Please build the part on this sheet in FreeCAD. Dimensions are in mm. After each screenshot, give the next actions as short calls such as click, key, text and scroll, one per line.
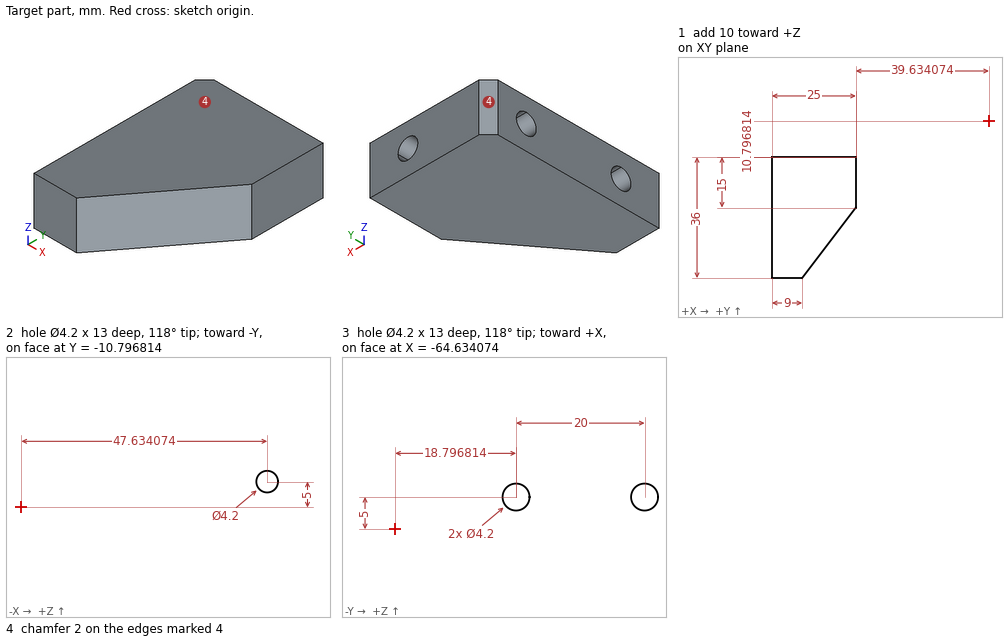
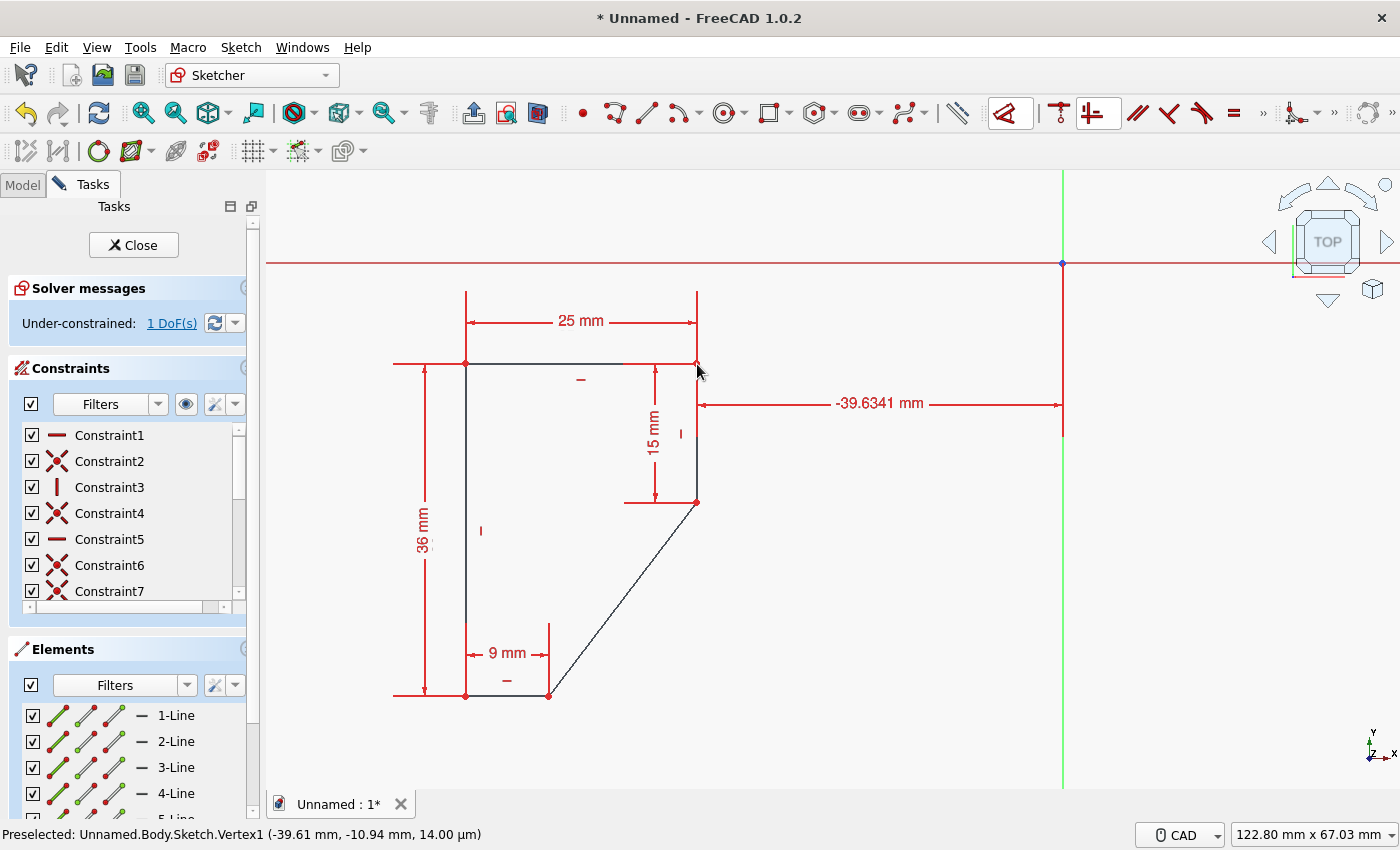
click(697, 364)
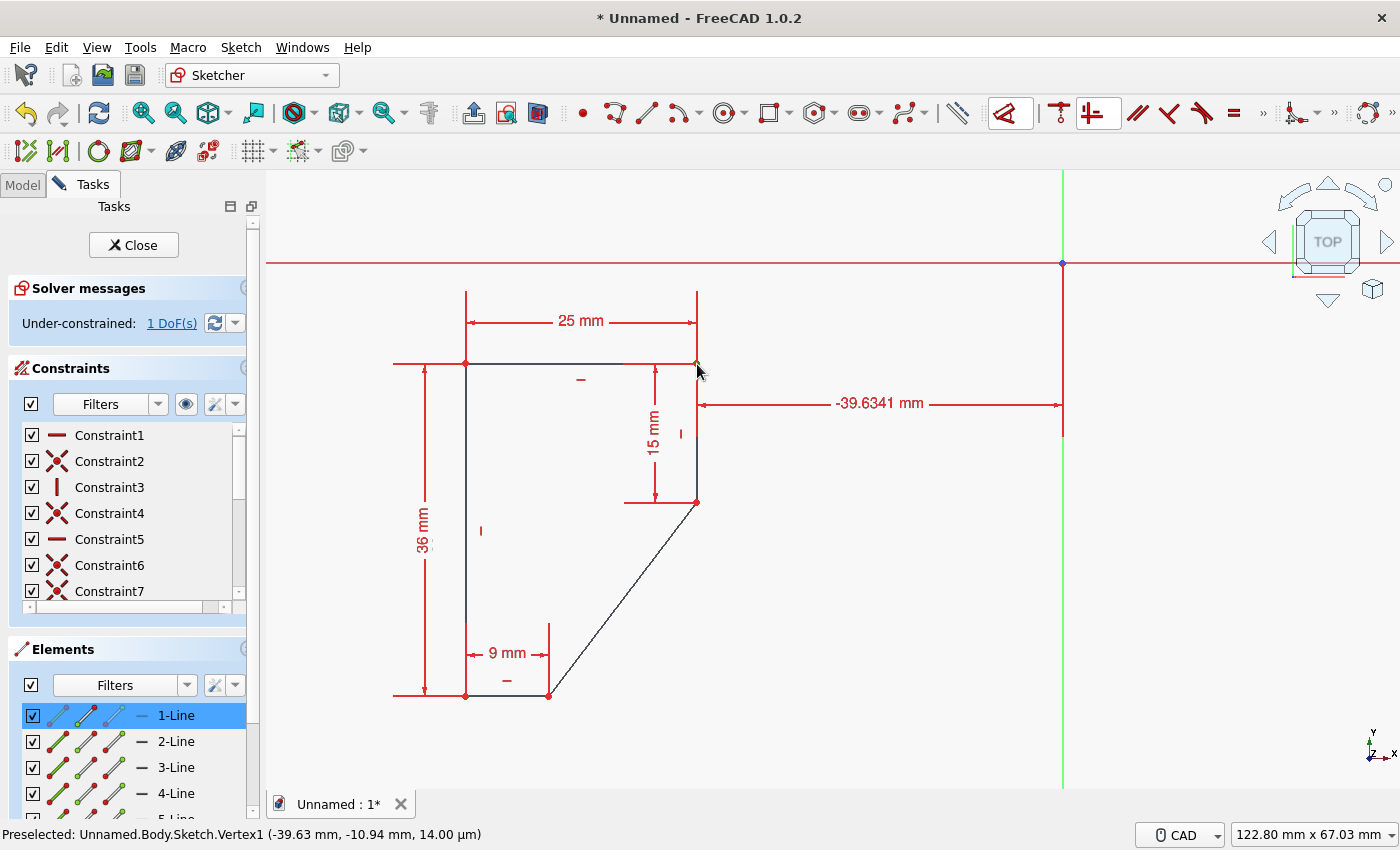
click(1028, 114)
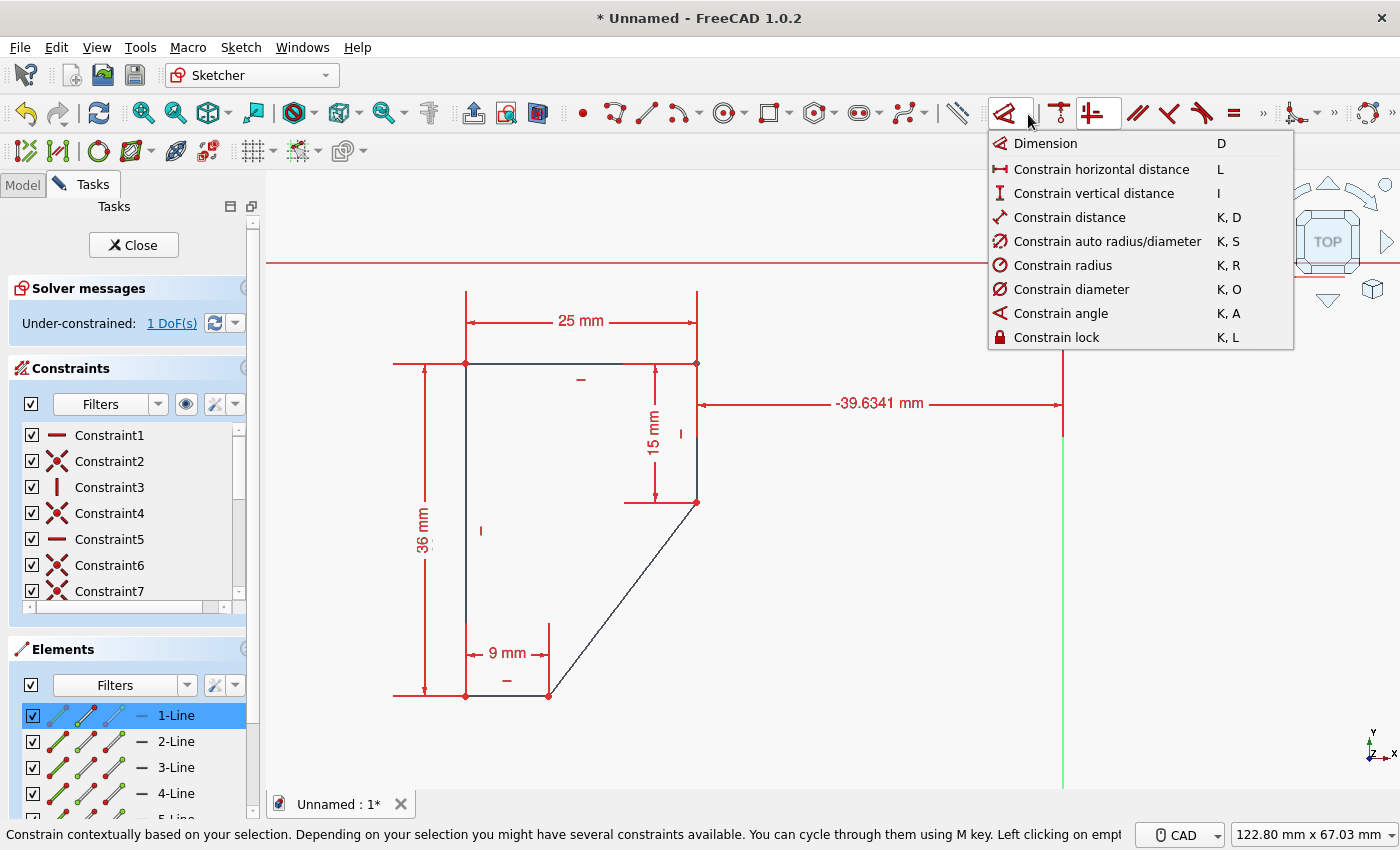
click(1141, 193)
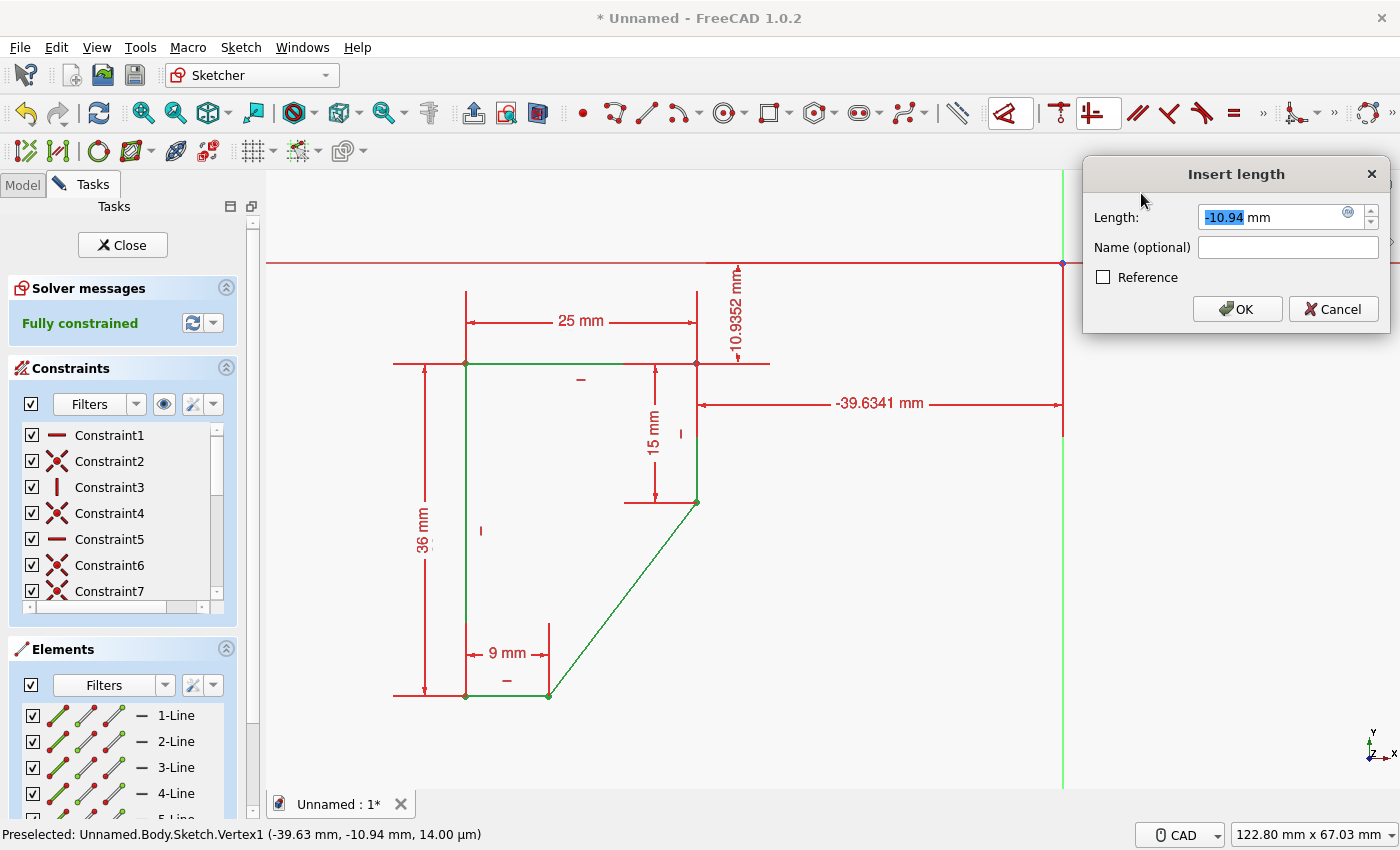
text(-10.796814)
key(Return)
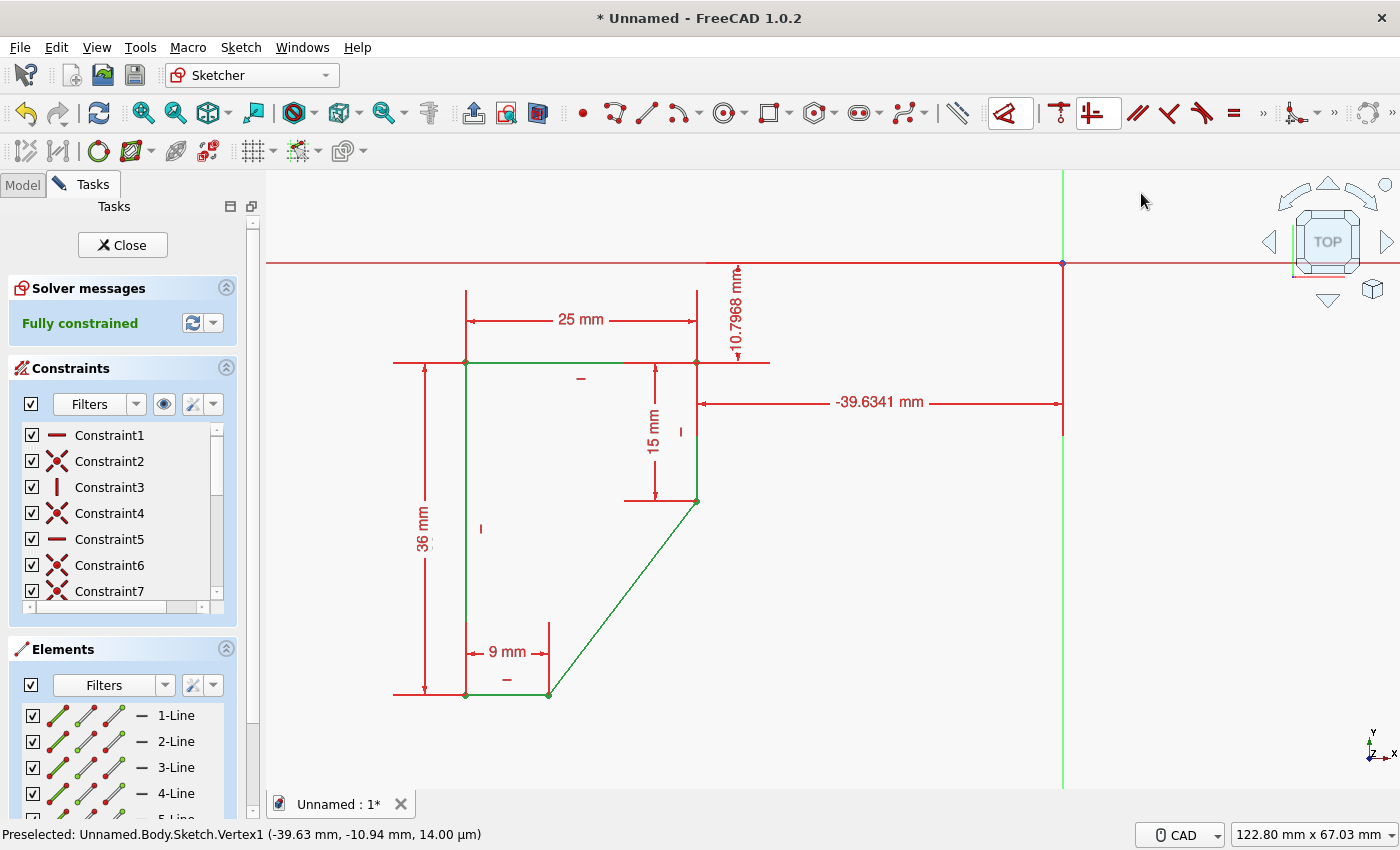
click(123, 245)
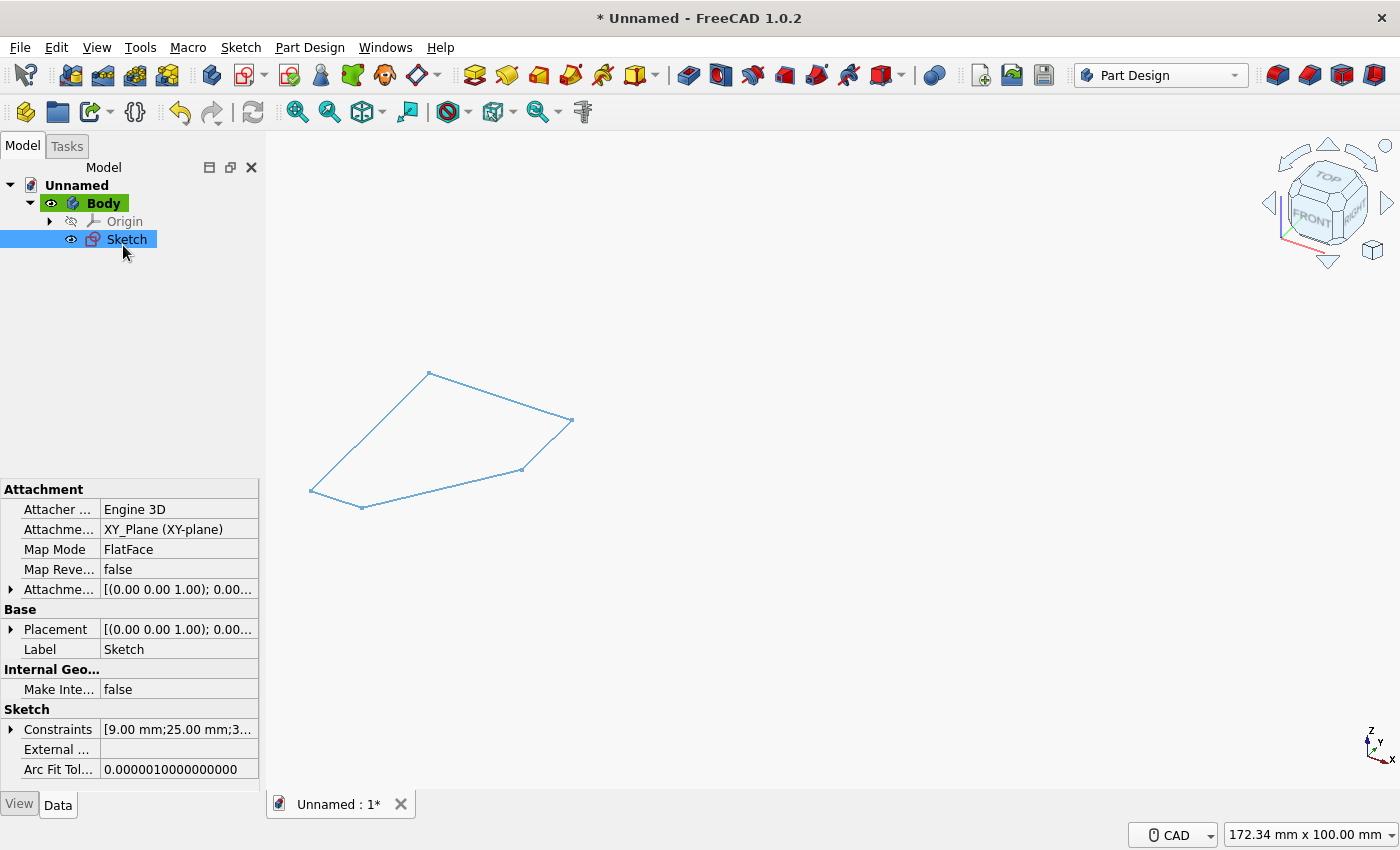
click(476, 76)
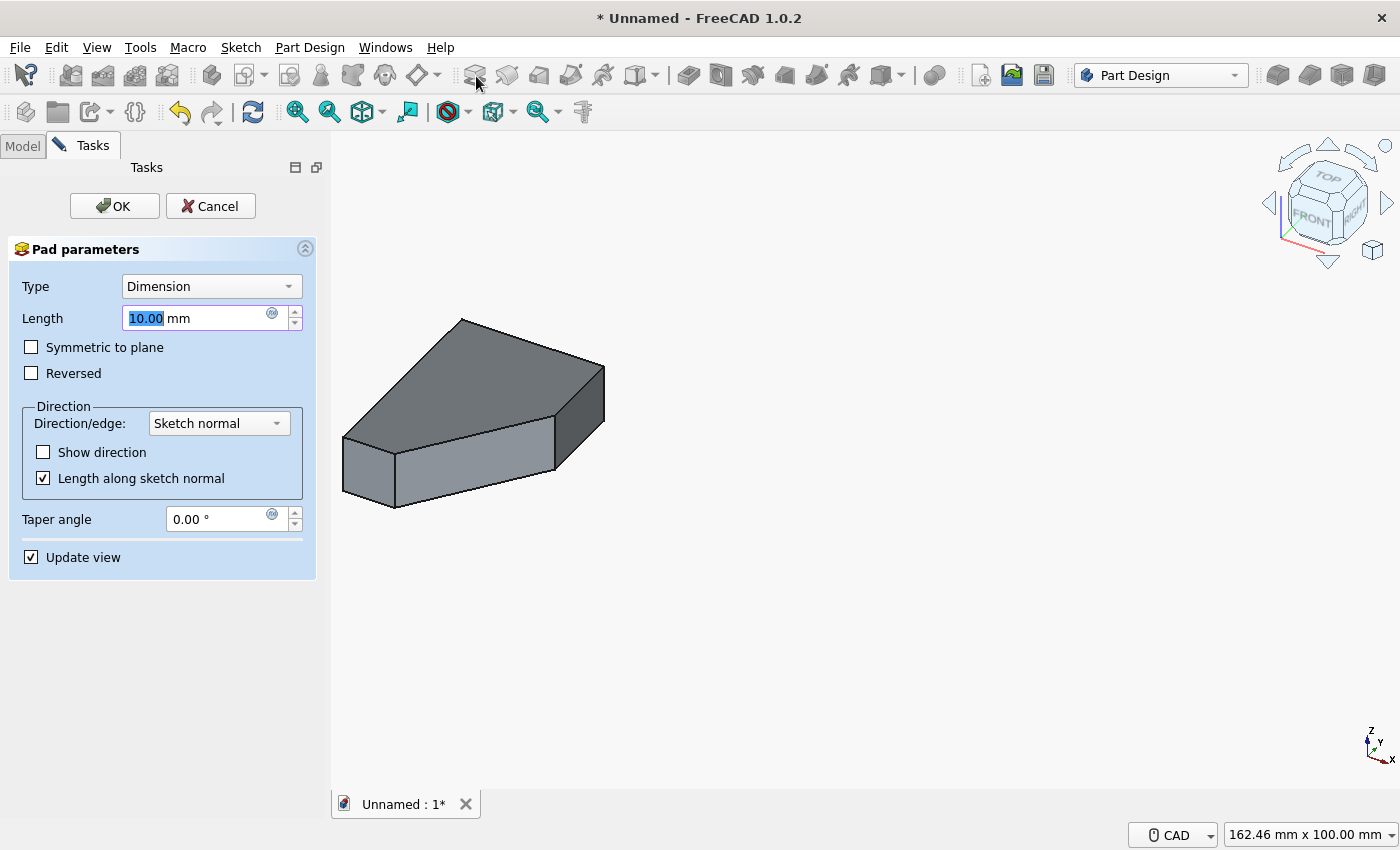
text(10)
key(Tab)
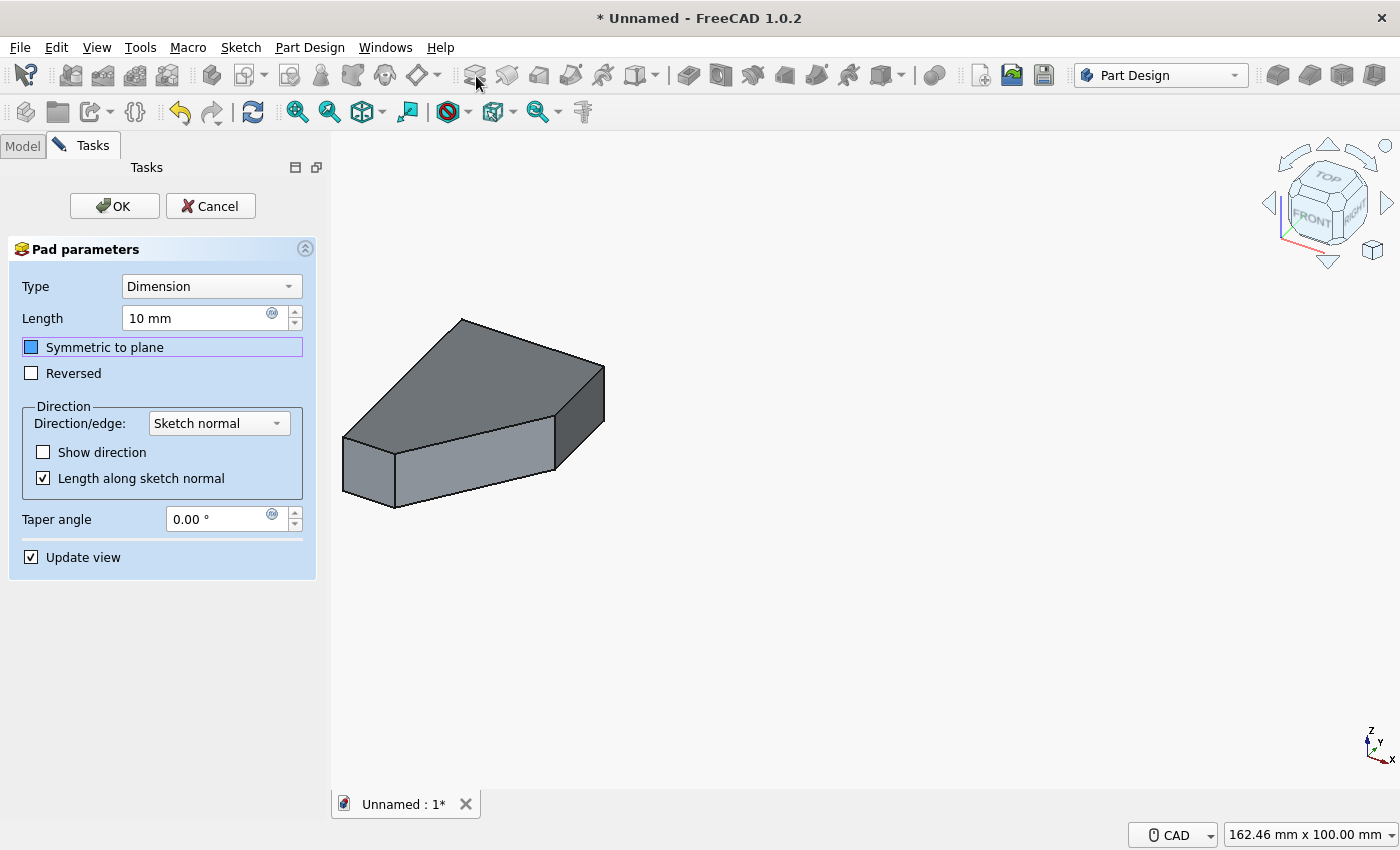
click(115, 206)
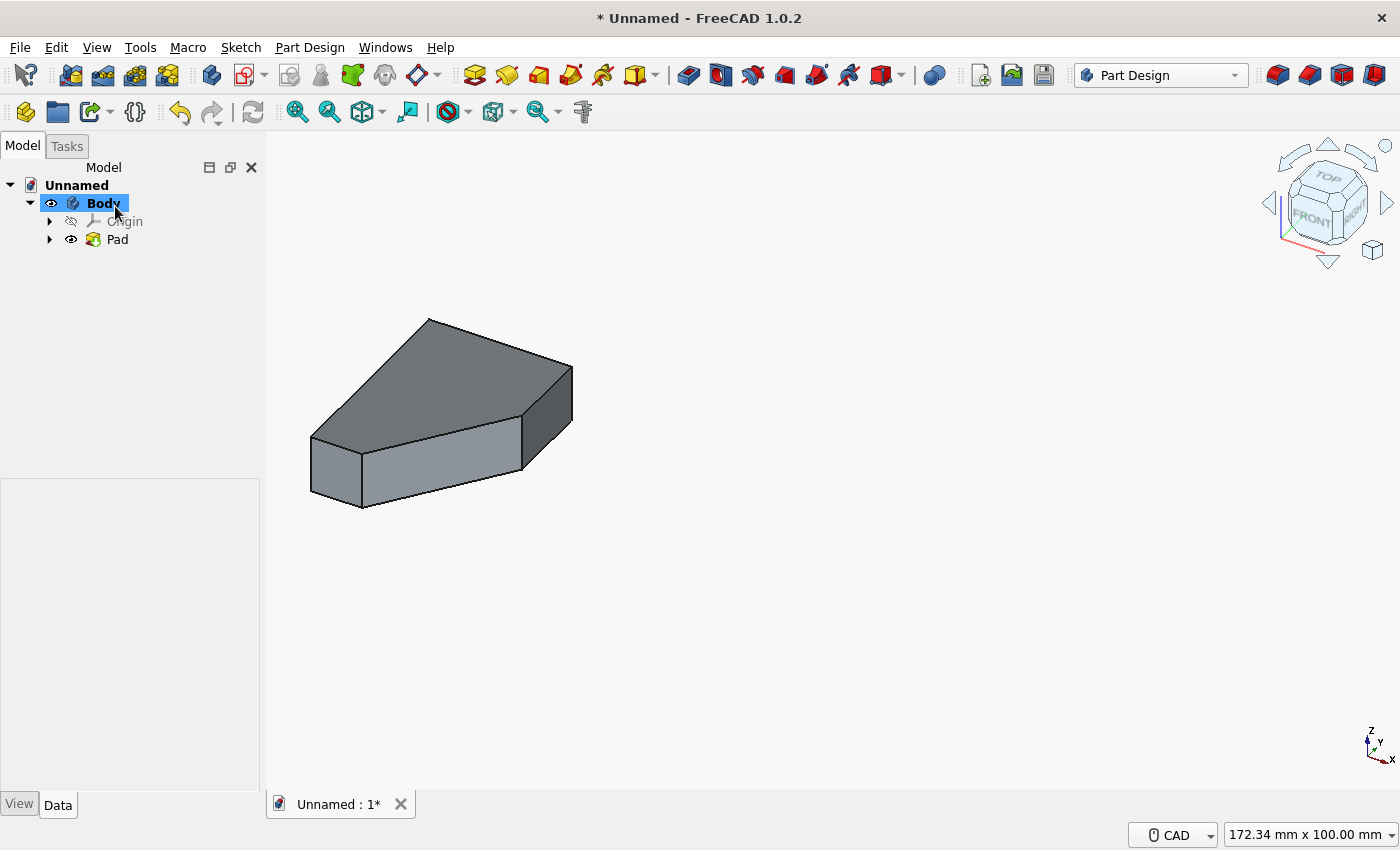
click(298, 112)